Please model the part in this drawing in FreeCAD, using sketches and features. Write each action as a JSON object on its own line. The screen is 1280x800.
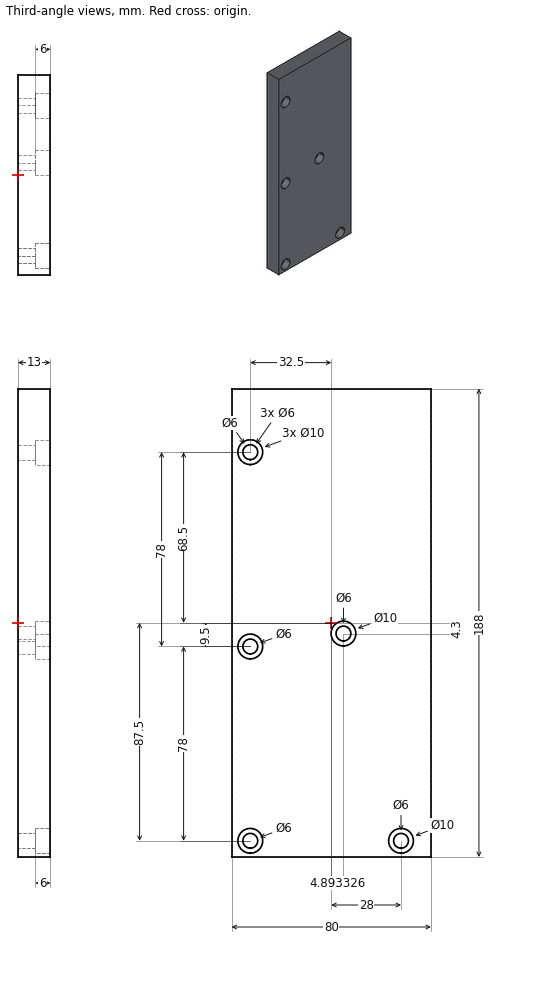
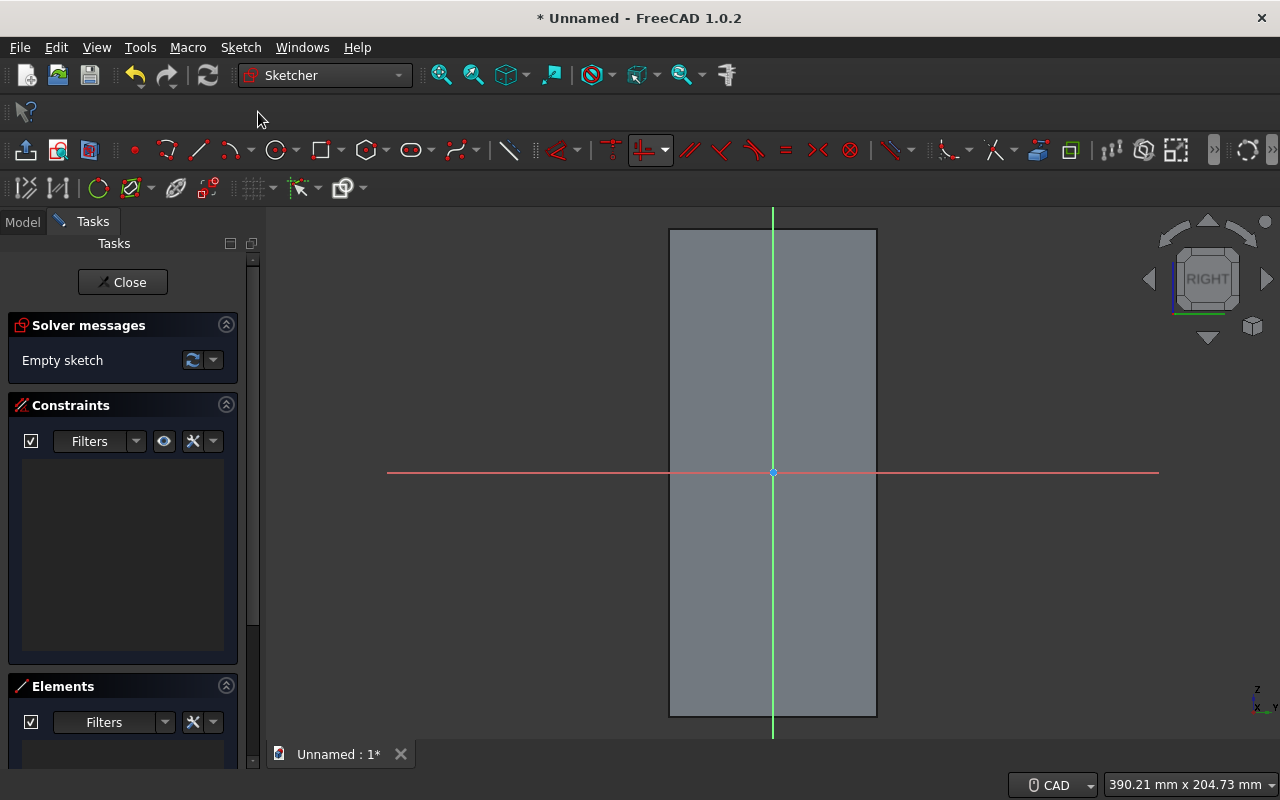
{"action": "scroll", "coordinate": [792, 485], "scroll_direction": "up", "scroll_amount": 13}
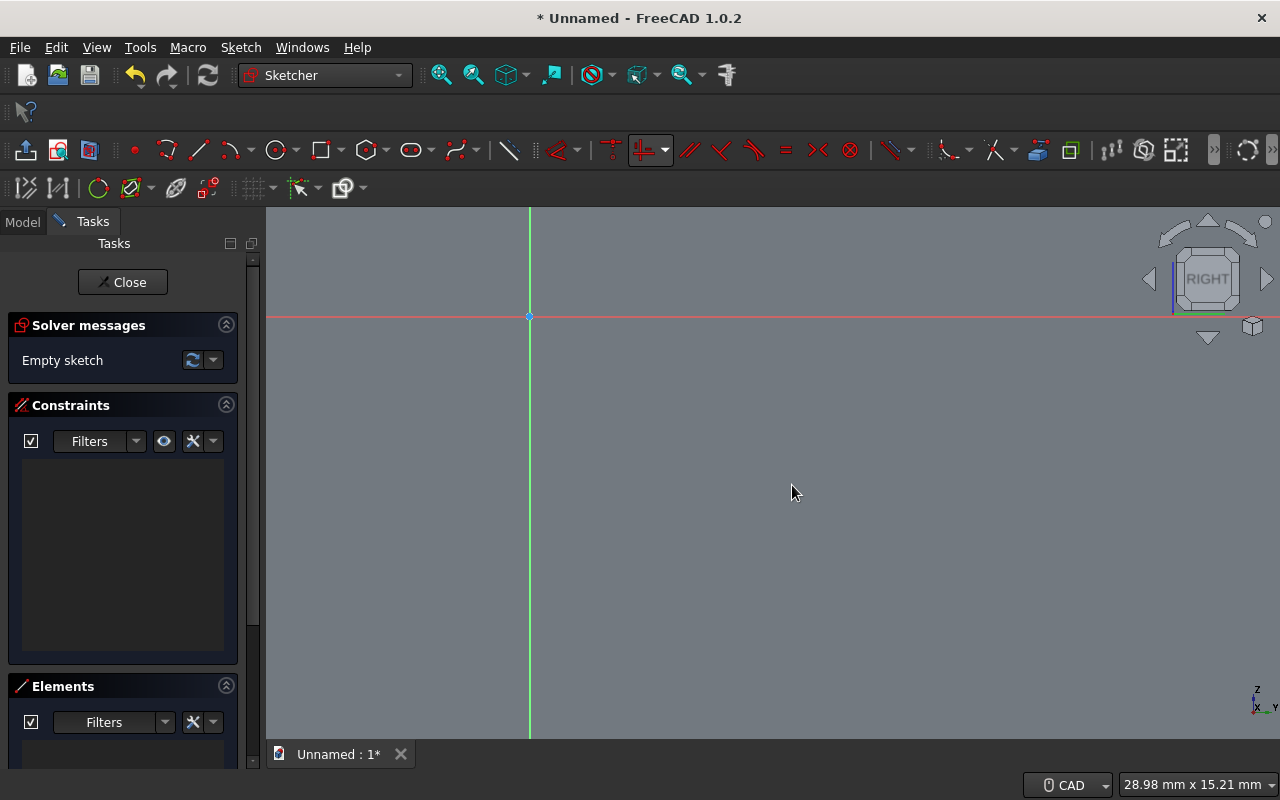
{"action": "left_click", "coordinate": [276, 150]}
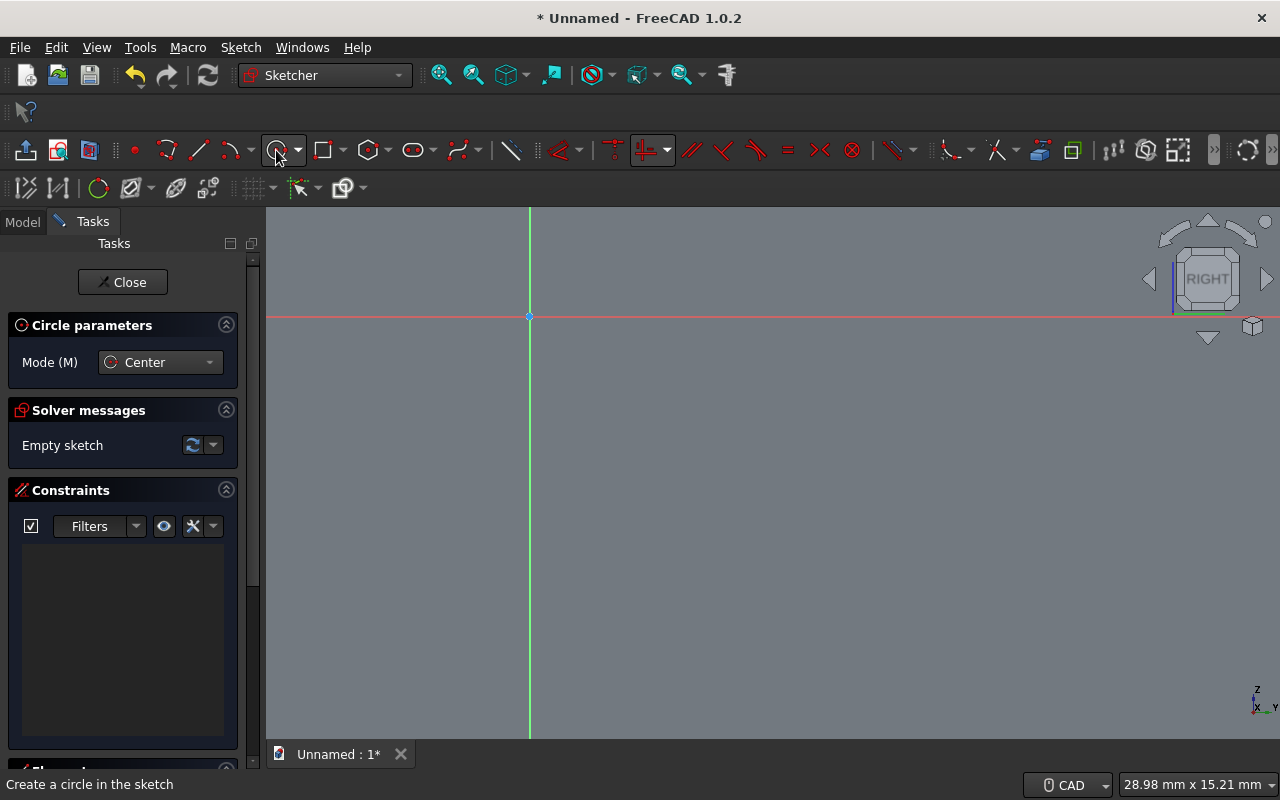
{"action": "left_click", "coordinate": [701, 467]}
{"action": "left_click", "coordinate": [825, 344]}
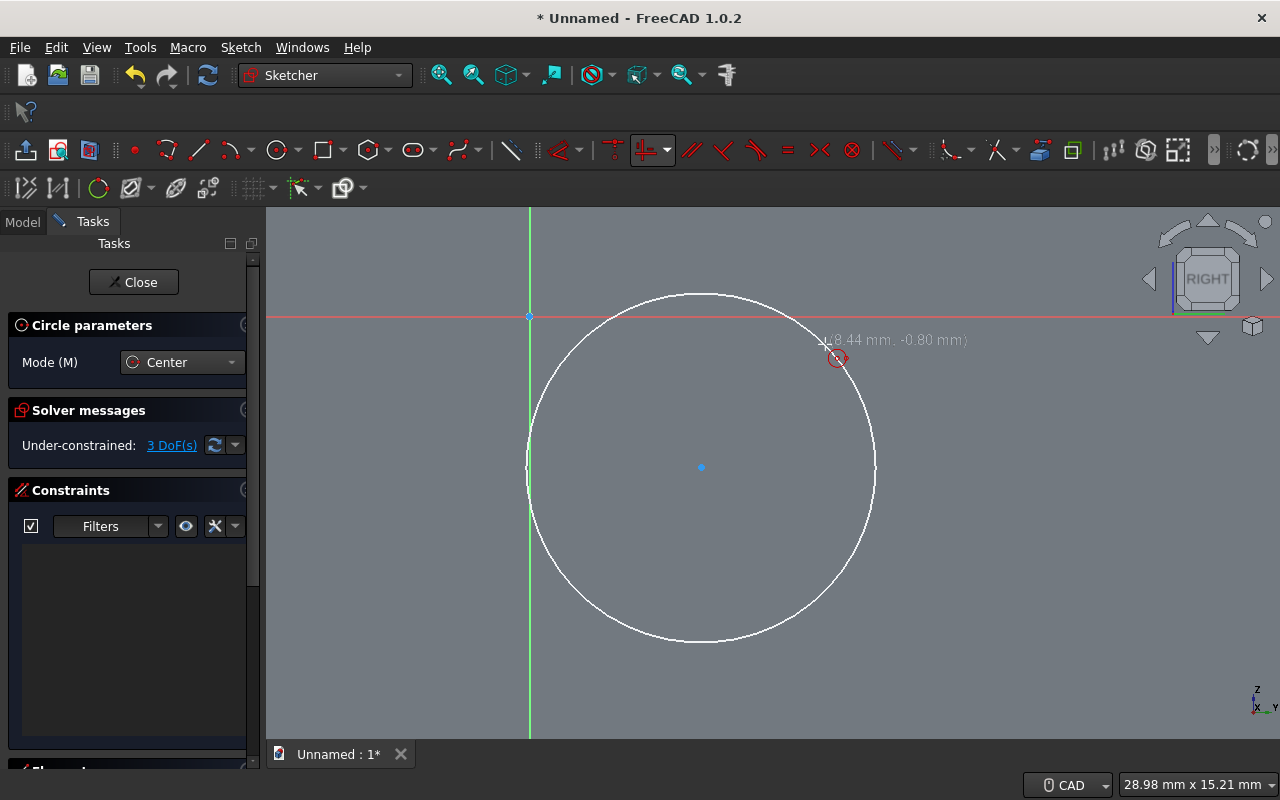
{"action": "left_click", "coordinate": [701, 468]}
{"action": "left_click", "coordinate": [775, 393]}
{"action": "key", "text": "Escape"}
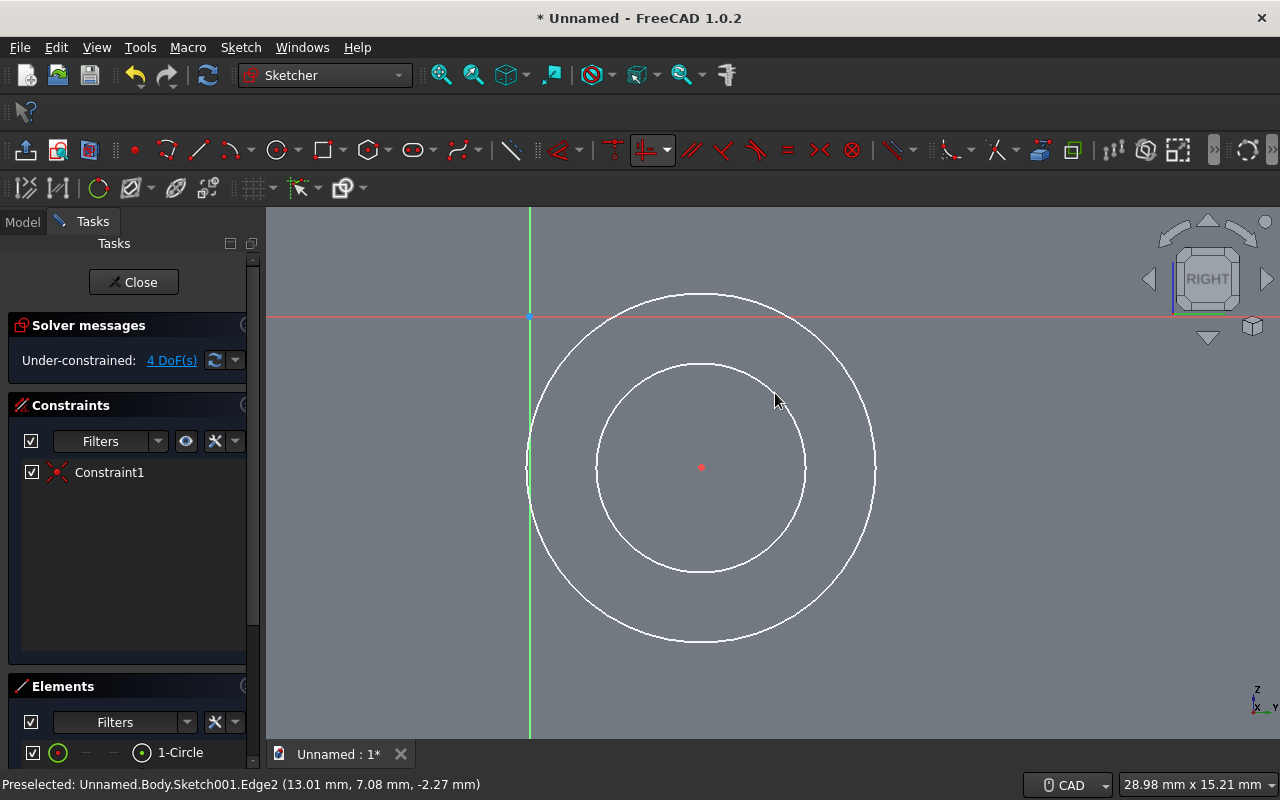
{"action": "left_click", "coordinate": [824, 344]}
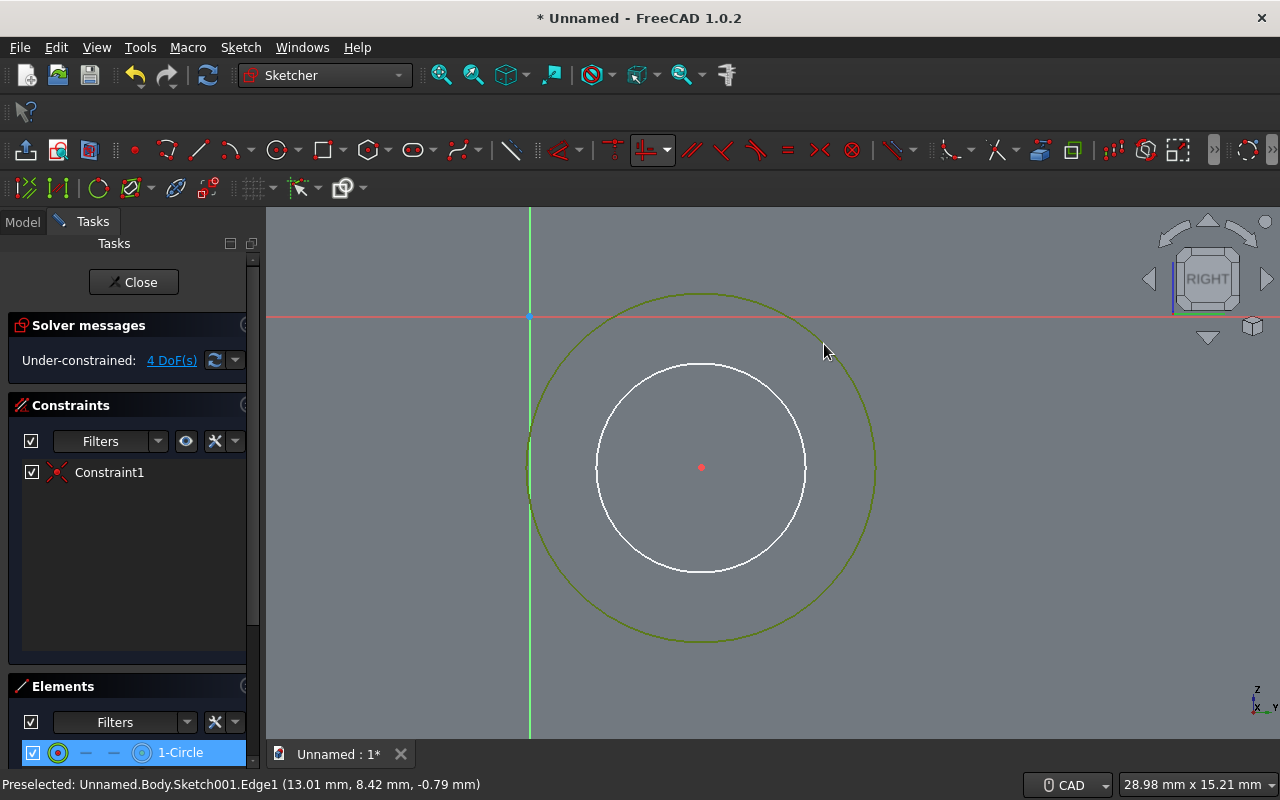
{"action": "left_click", "coordinate": [582, 150]}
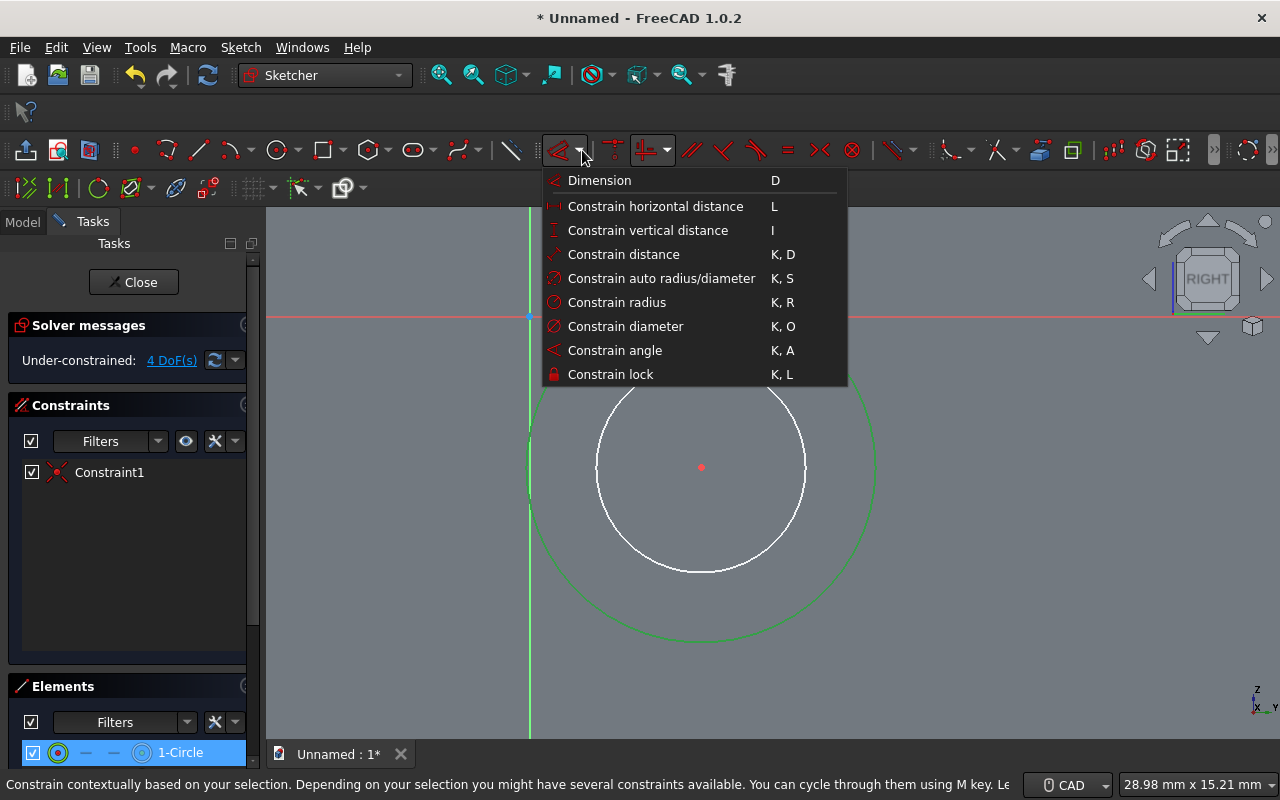
{"action": "left_click", "coordinate": [695, 326]}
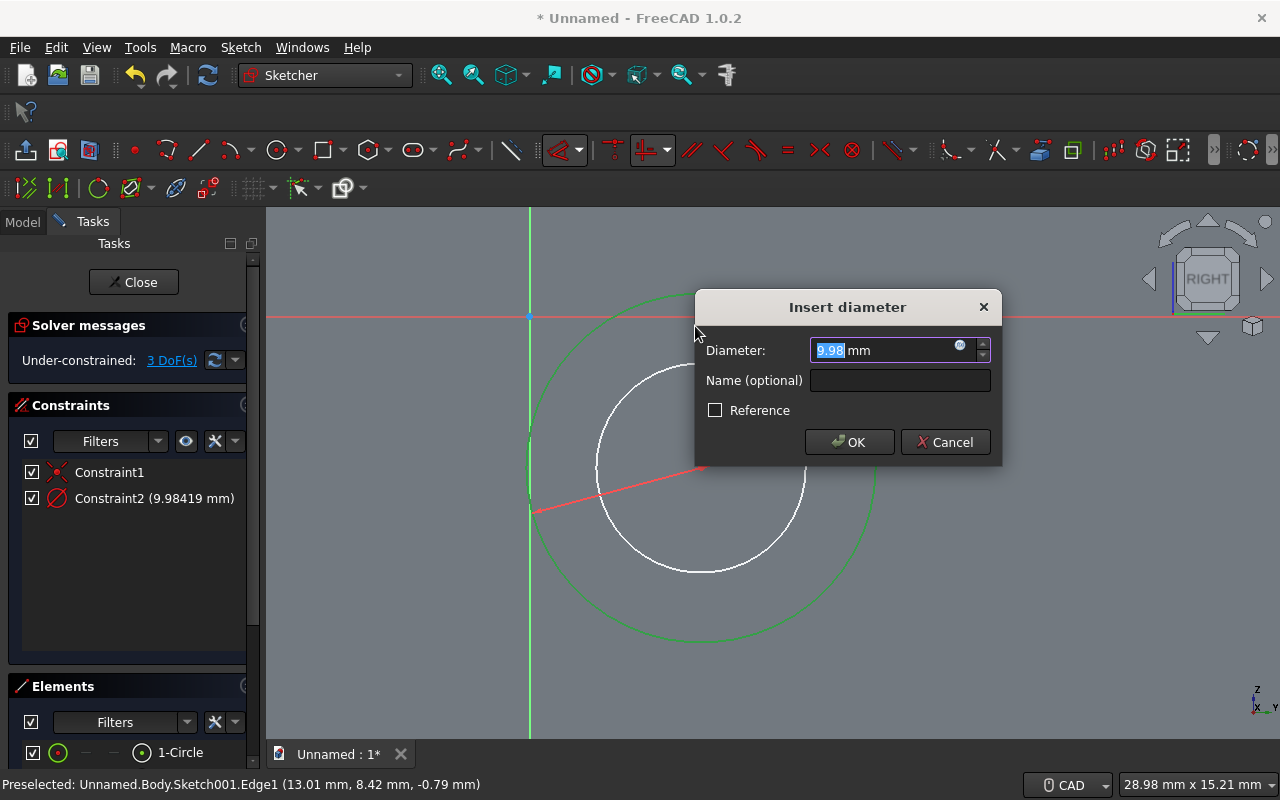
{"action": "type", "text": "10"}
{"action": "key", "text": "Return"}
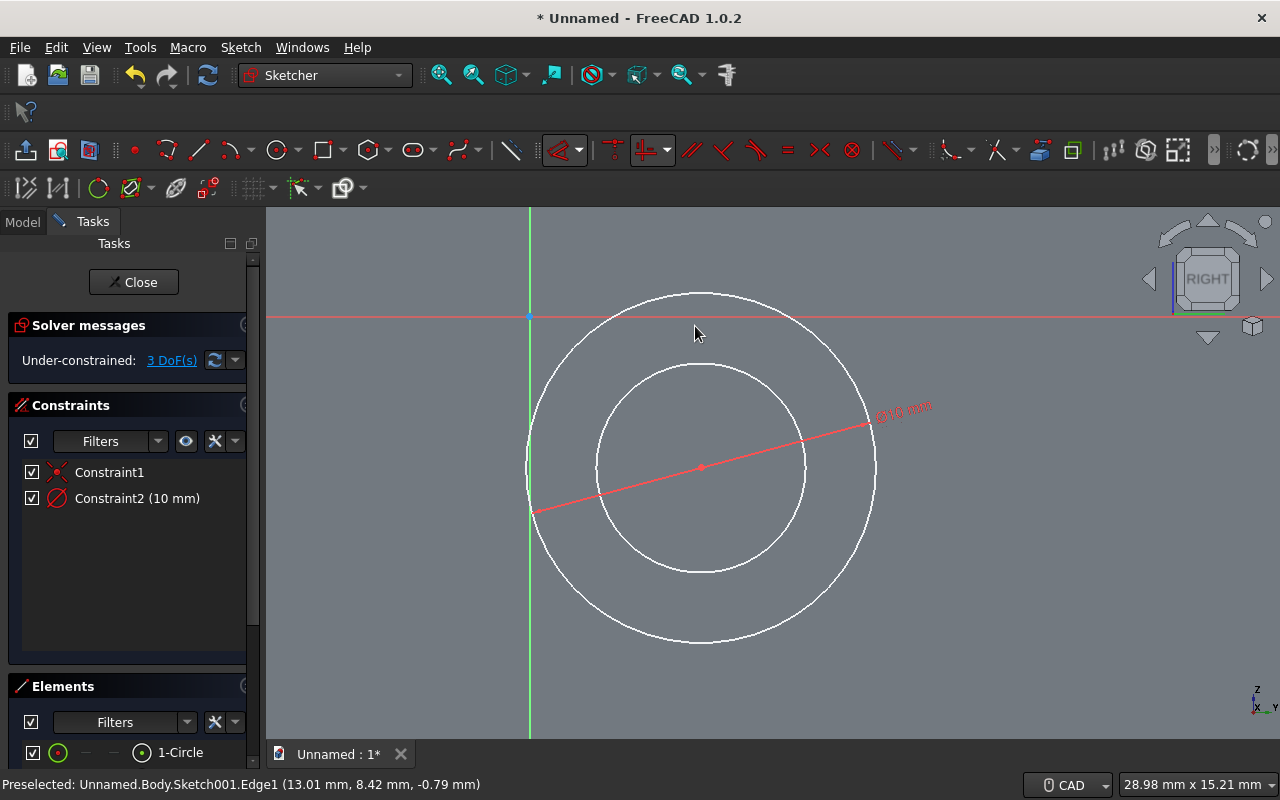
{"action": "left_click", "coordinate": [775, 394]}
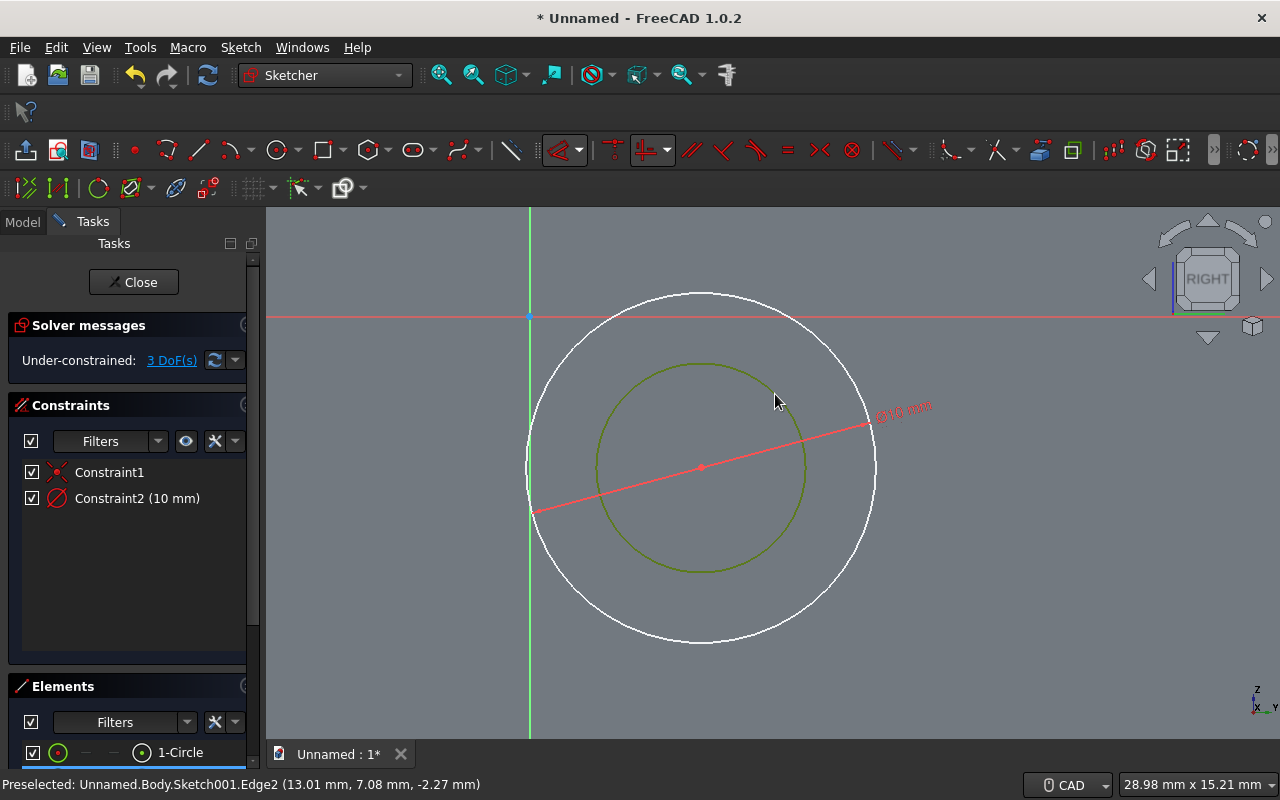
{"action": "key", "text": "k o"}